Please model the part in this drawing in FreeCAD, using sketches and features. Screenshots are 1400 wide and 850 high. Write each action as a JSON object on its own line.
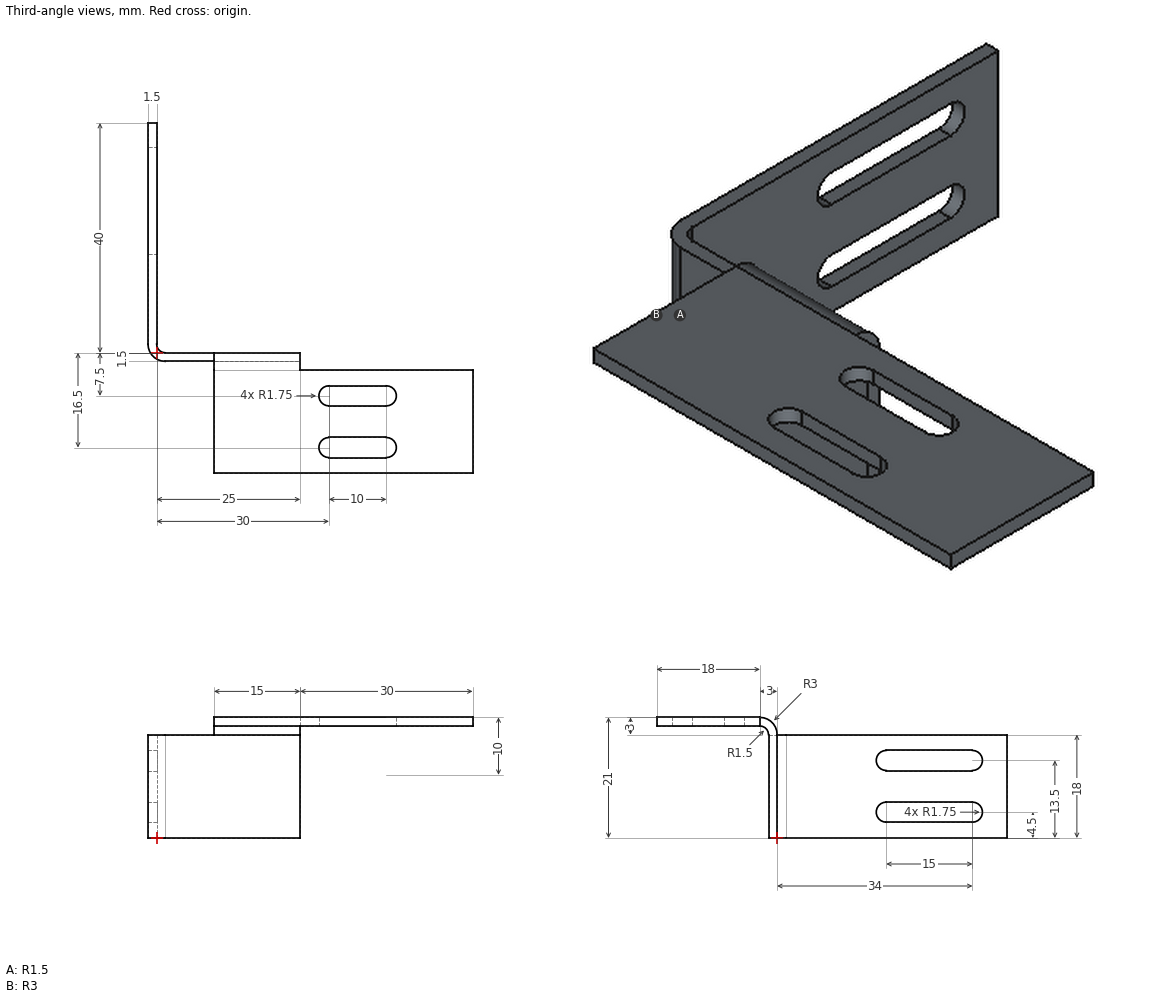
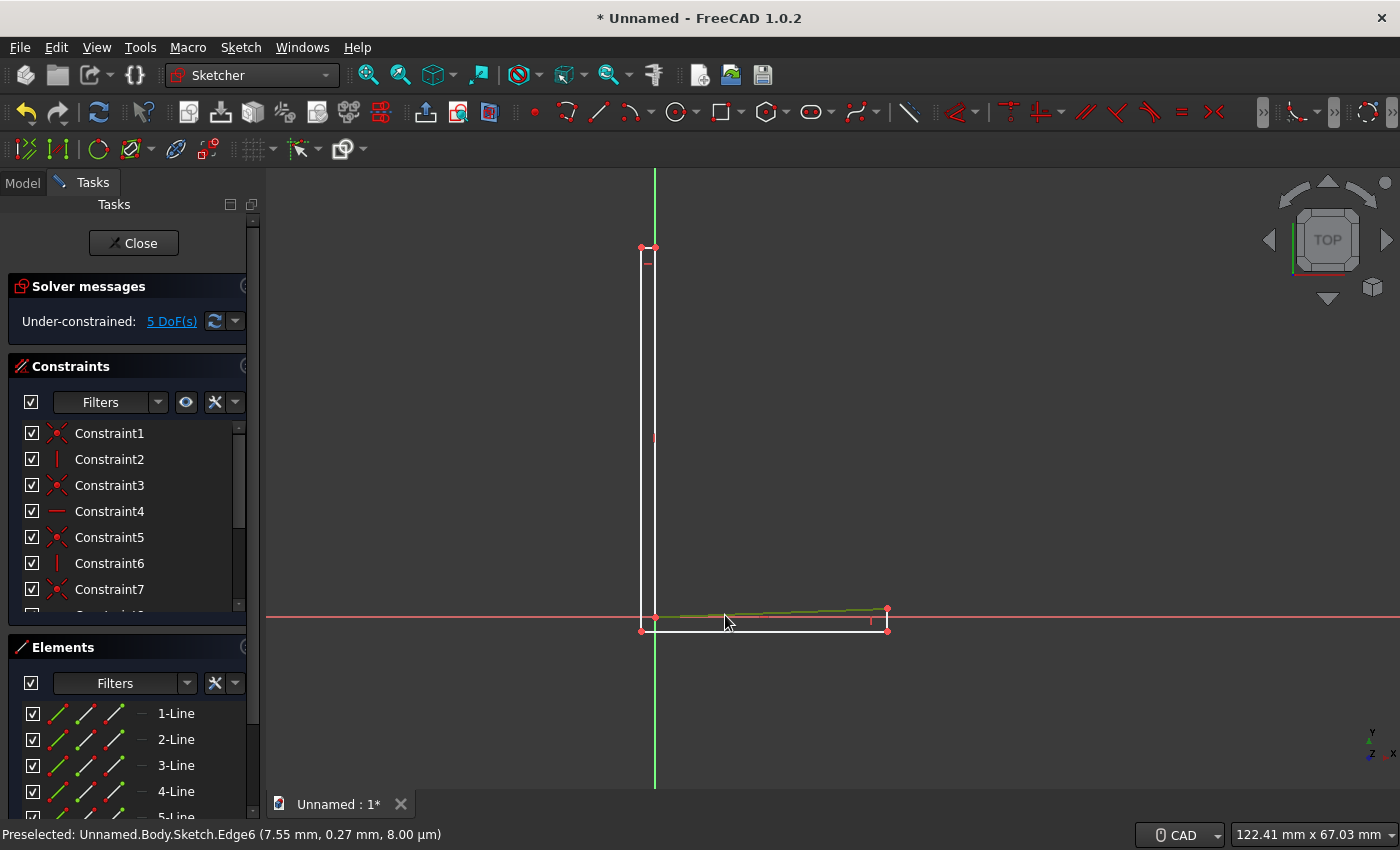
{"action": "key", "text": "h"}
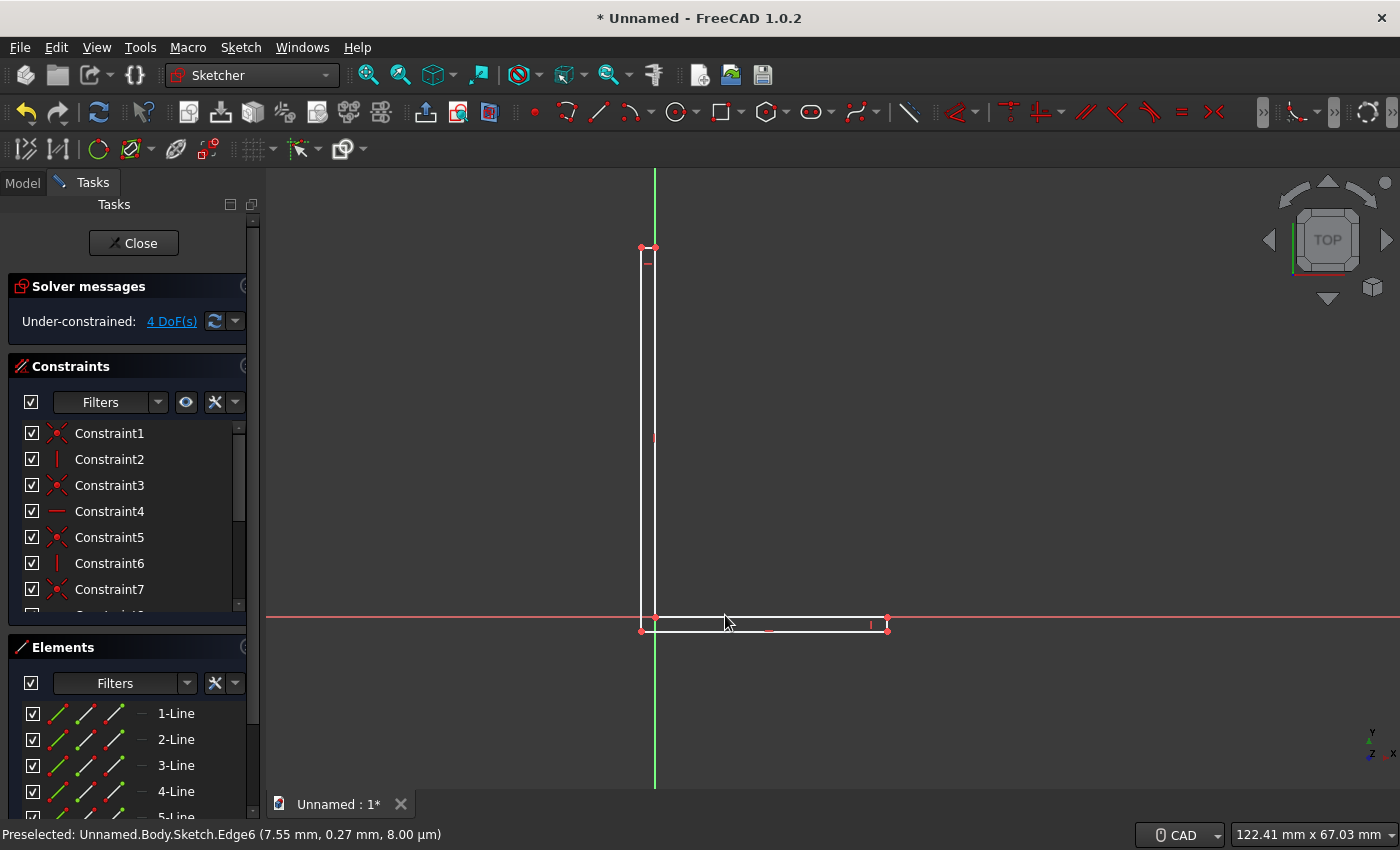
{"action": "key", "text": "d"}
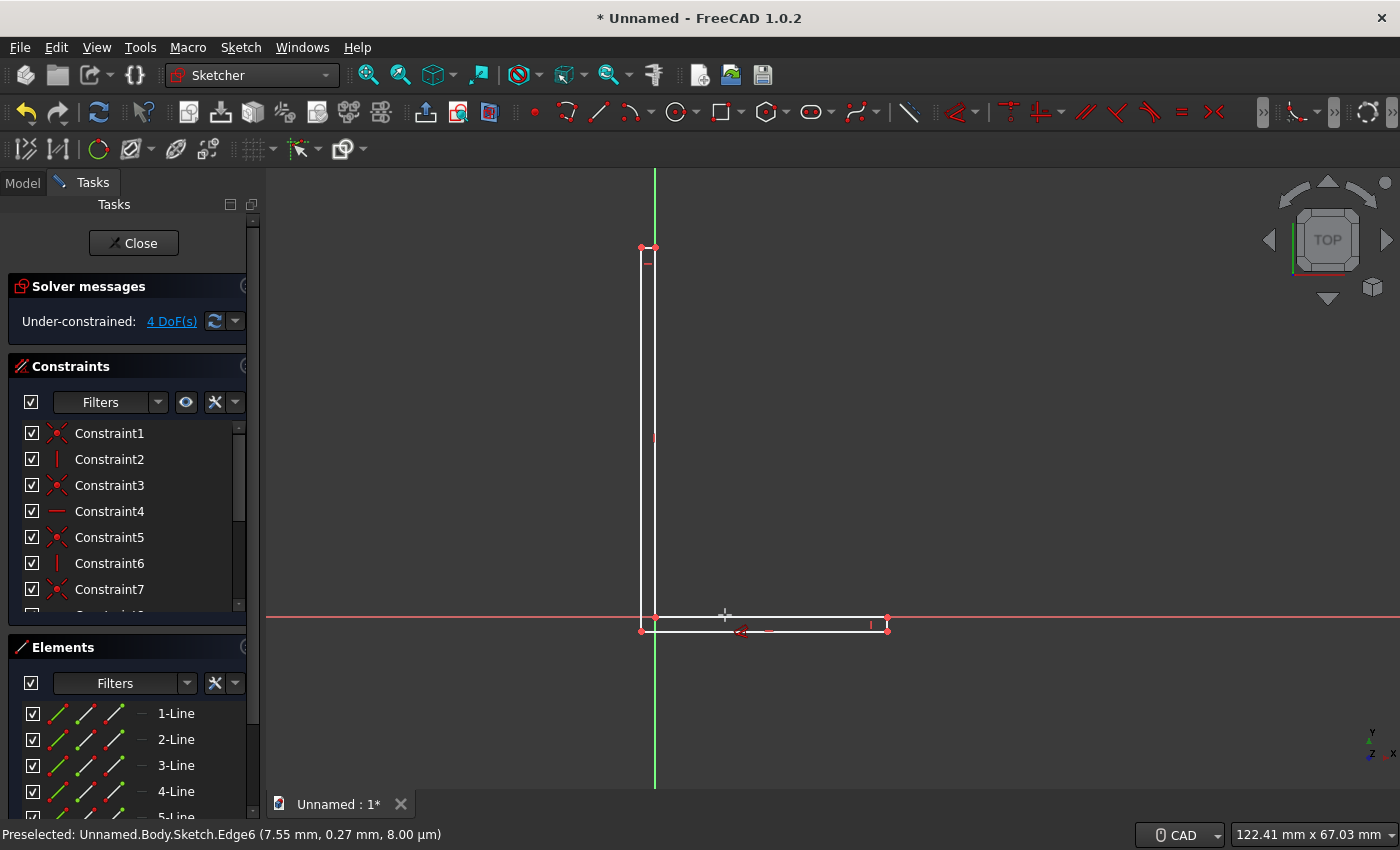
{"action": "left_click", "coordinate": [655, 507]}
{"action": "left_click", "coordinate": [621, 433]}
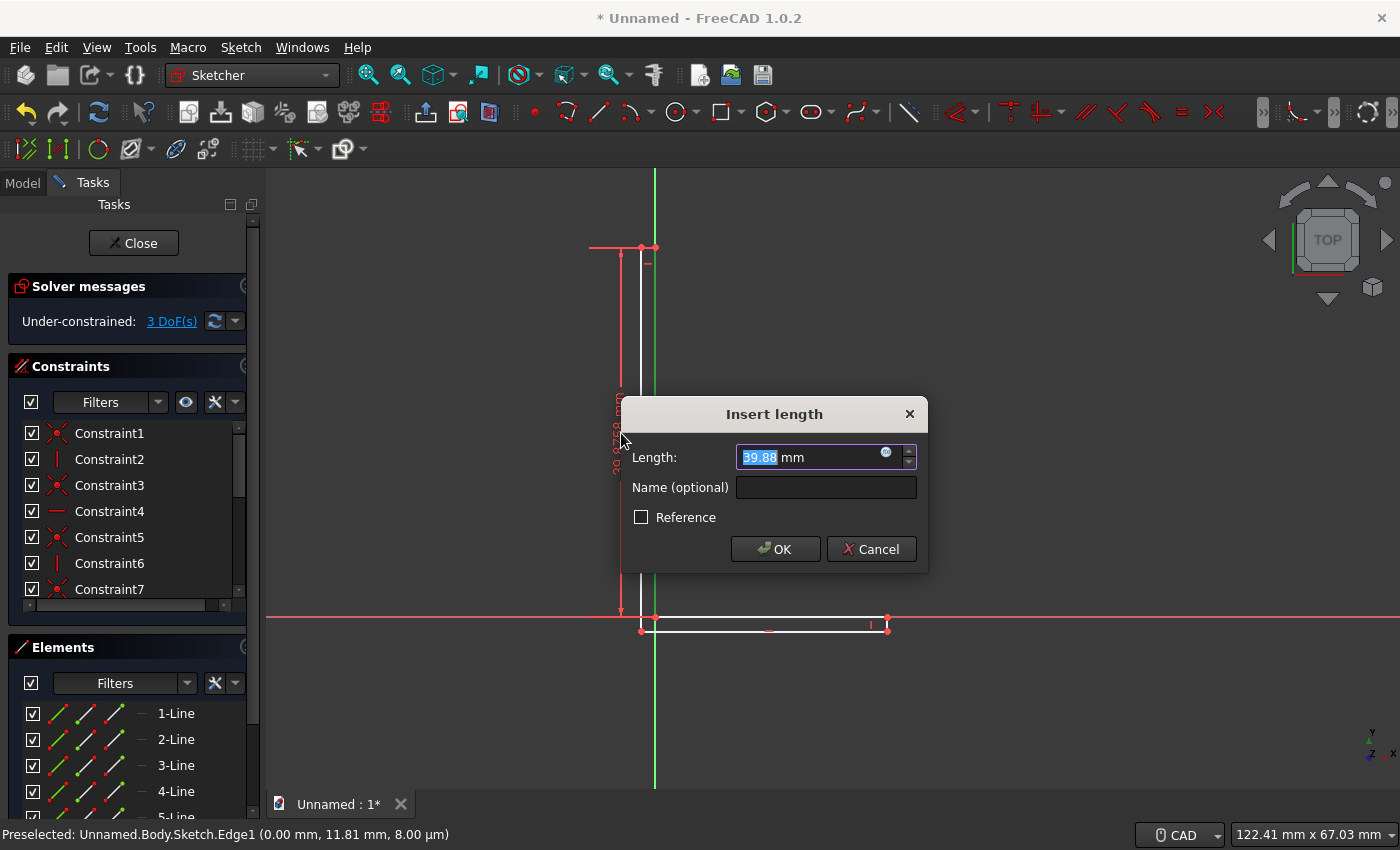
{"action": "type", "text": "40"}
{"action": "key", "text": "Return"}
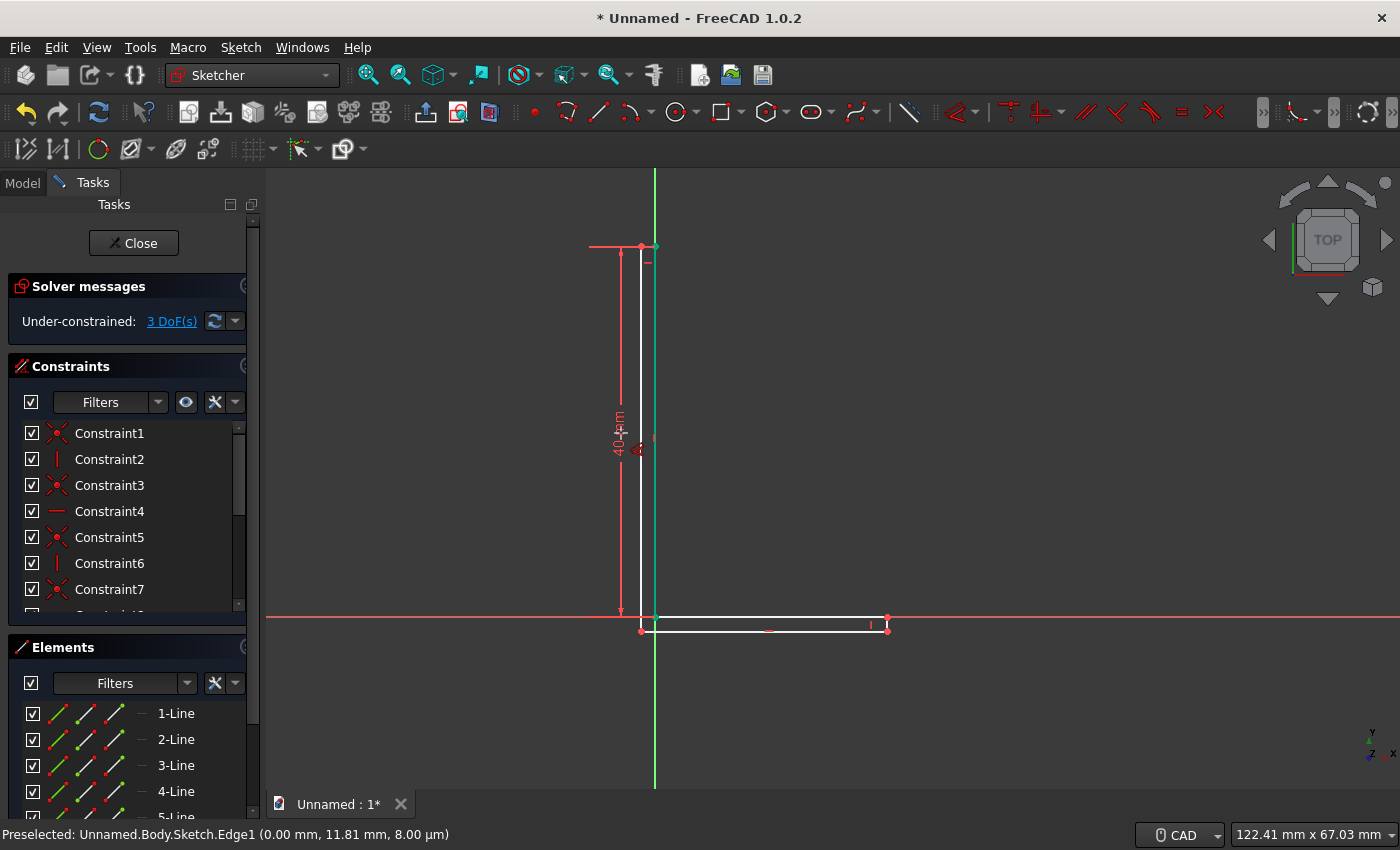
{"action": "left_click", "coordinate": [817, 617]}
{"action": "left_click", "coordinate": [771, 651]}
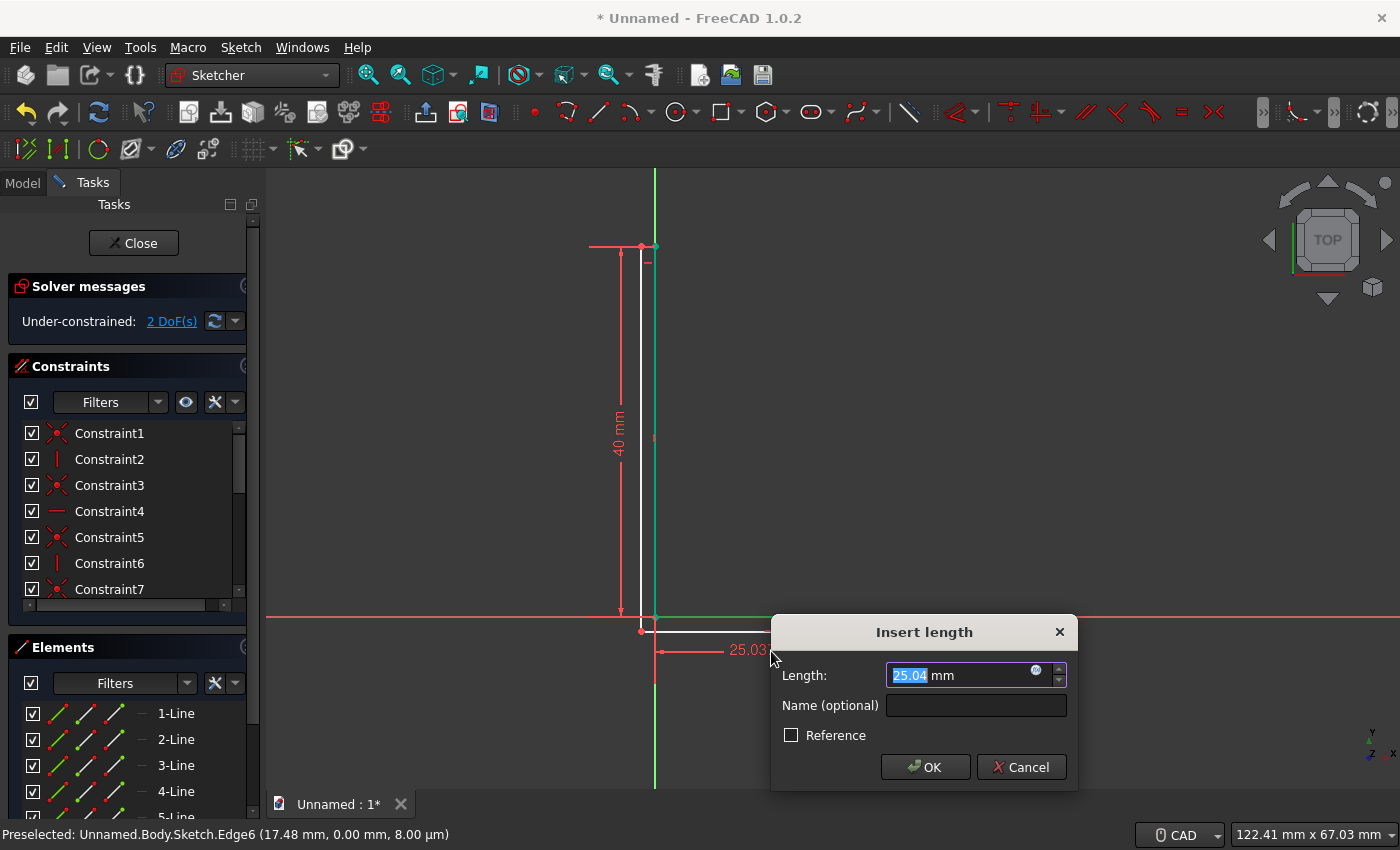
{"action": "type", "text": "25"}
{"action": "key", "text": "Return"}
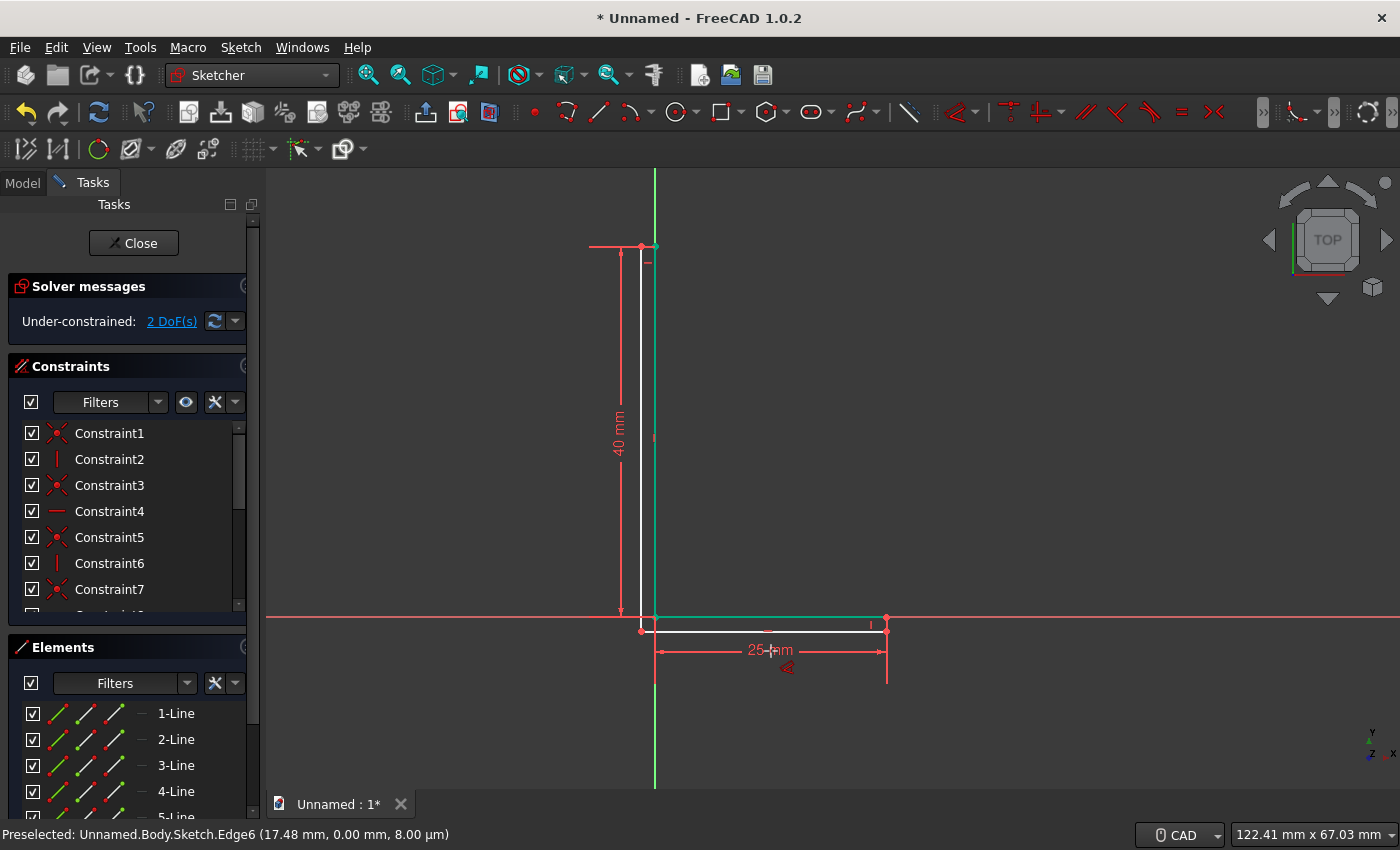
{"action": "scroll", "coordinate": [648, 247], "scroll_direction": "up", "scroll_amount": 6}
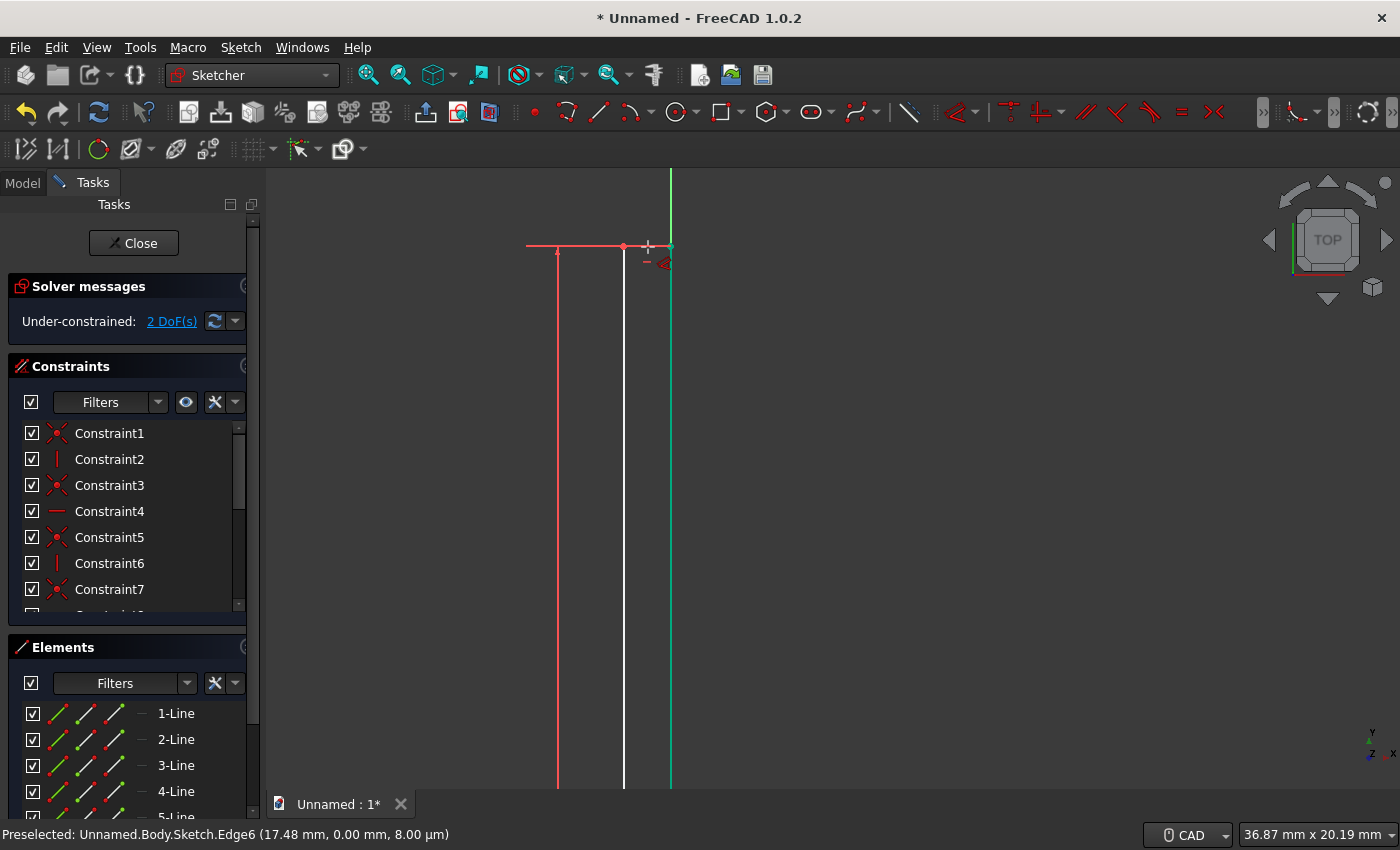
{"action": "left_click", "coordinate": [647, 246]}
{"action": "left_click", "coordinate": [647, 212]}